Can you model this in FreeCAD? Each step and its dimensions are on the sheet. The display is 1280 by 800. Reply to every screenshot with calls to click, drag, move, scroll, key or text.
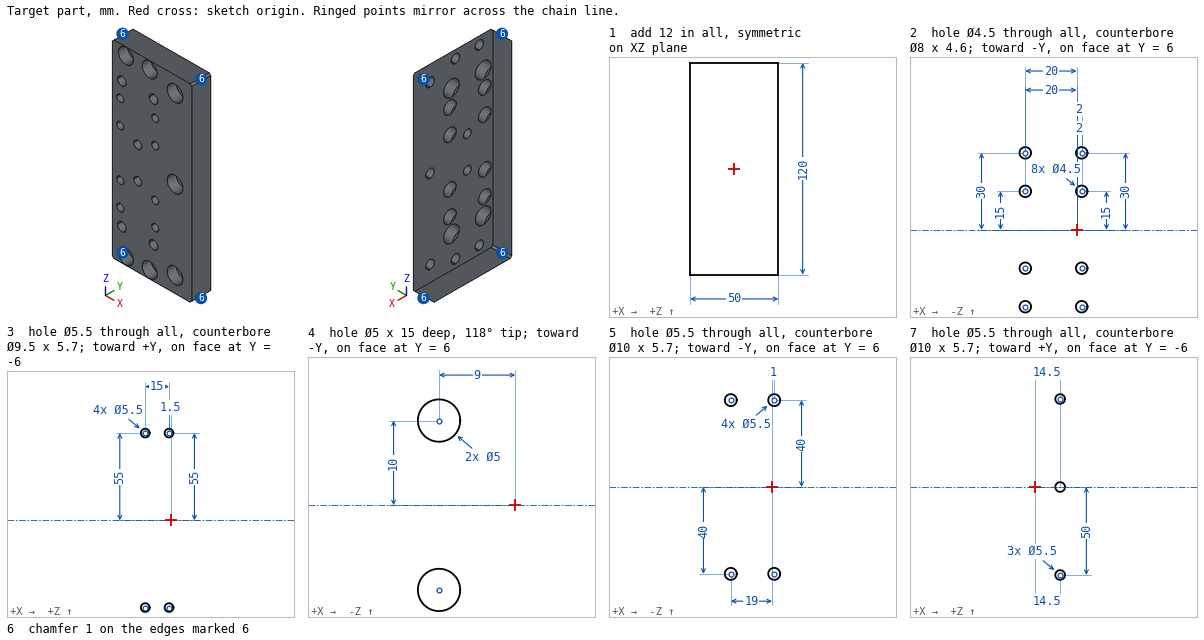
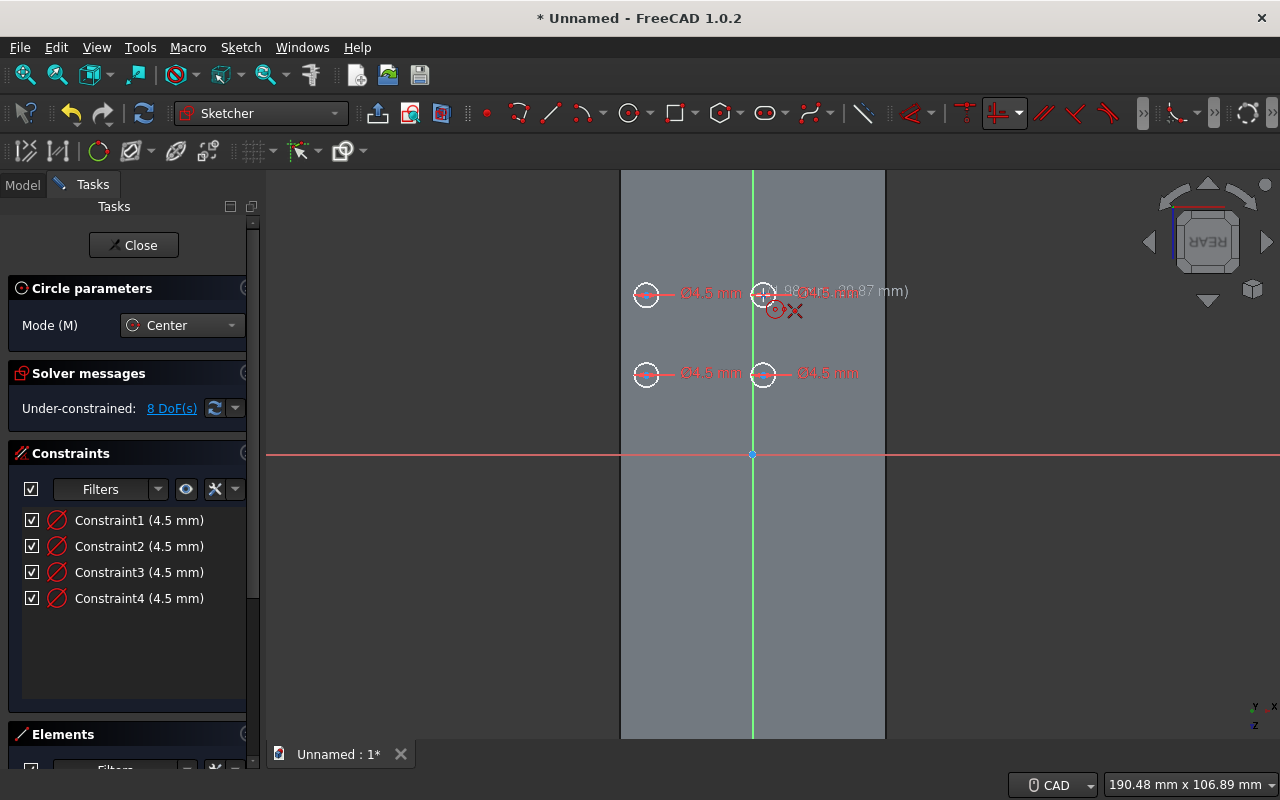
scroll(646, 534, up, 4)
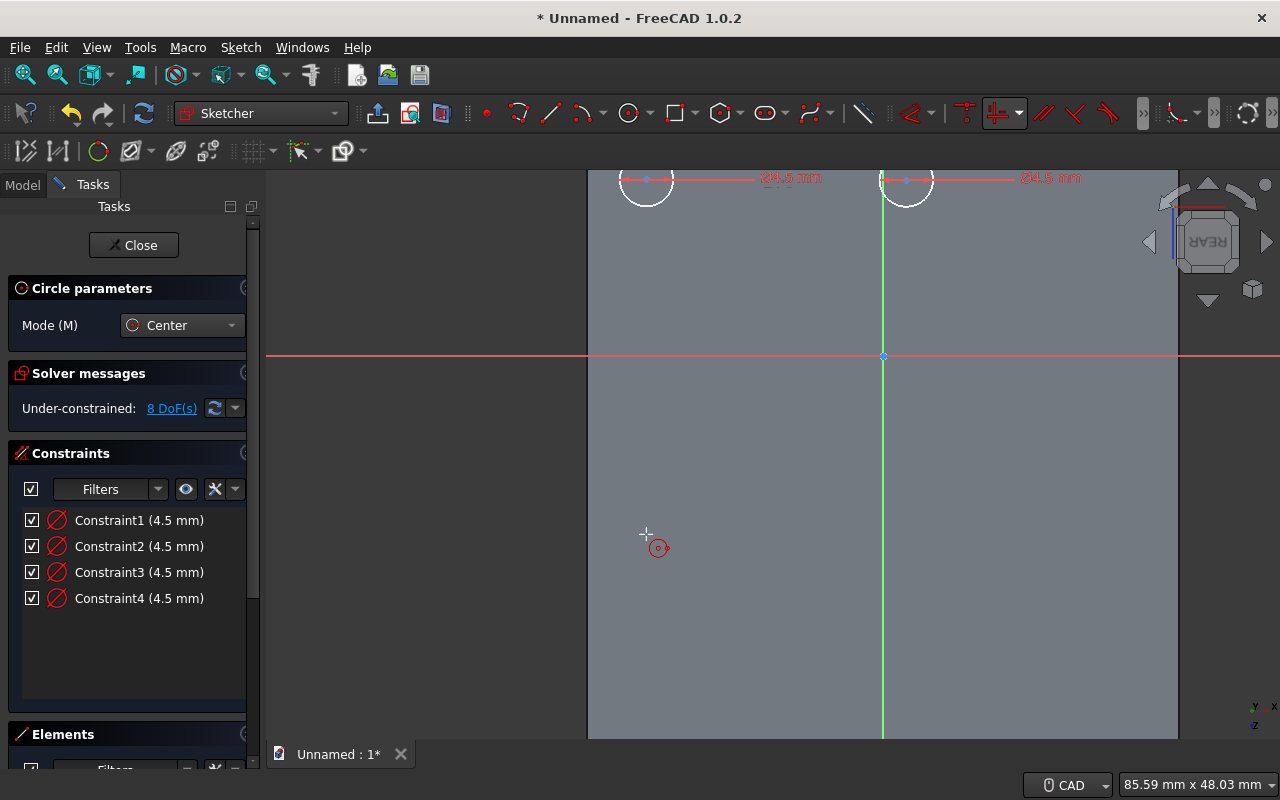
click(646, 534)
move(665, 515)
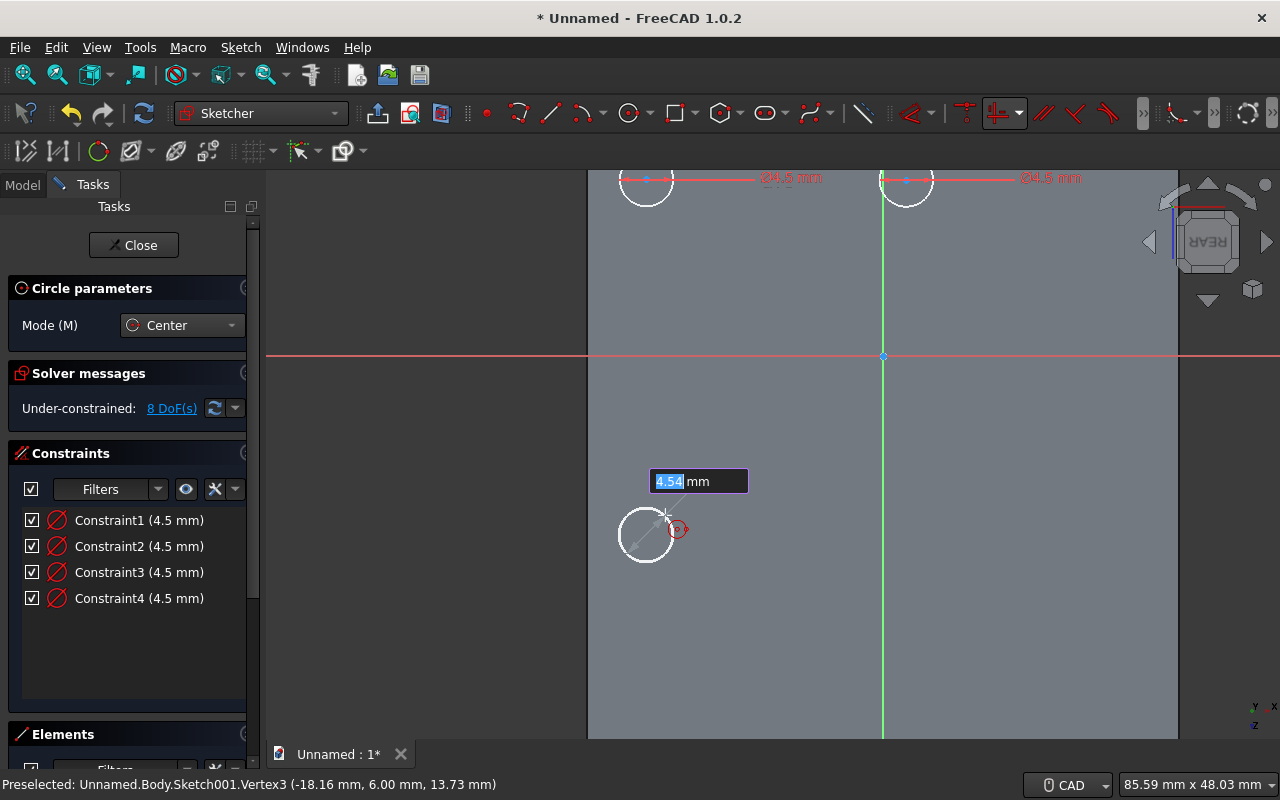
text(4.5)
key(Return)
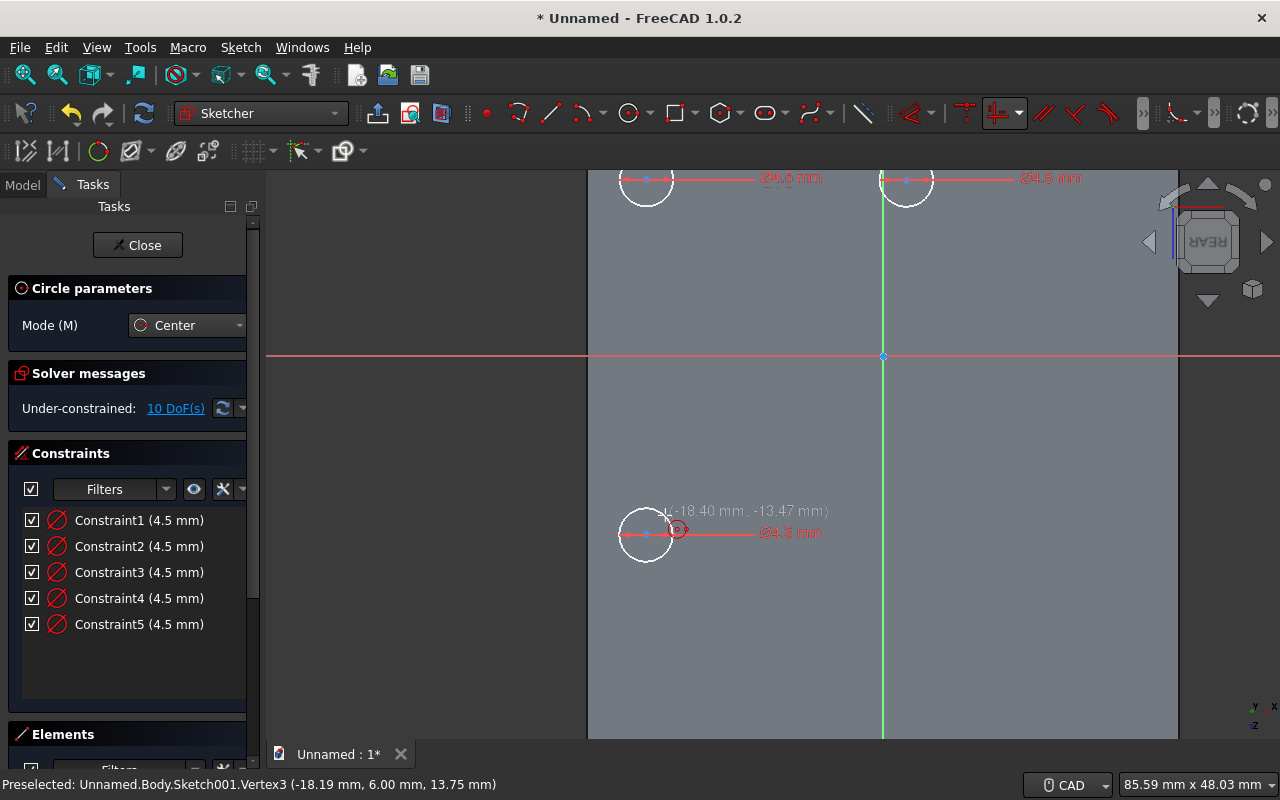
scroll(646, 535, down, 4)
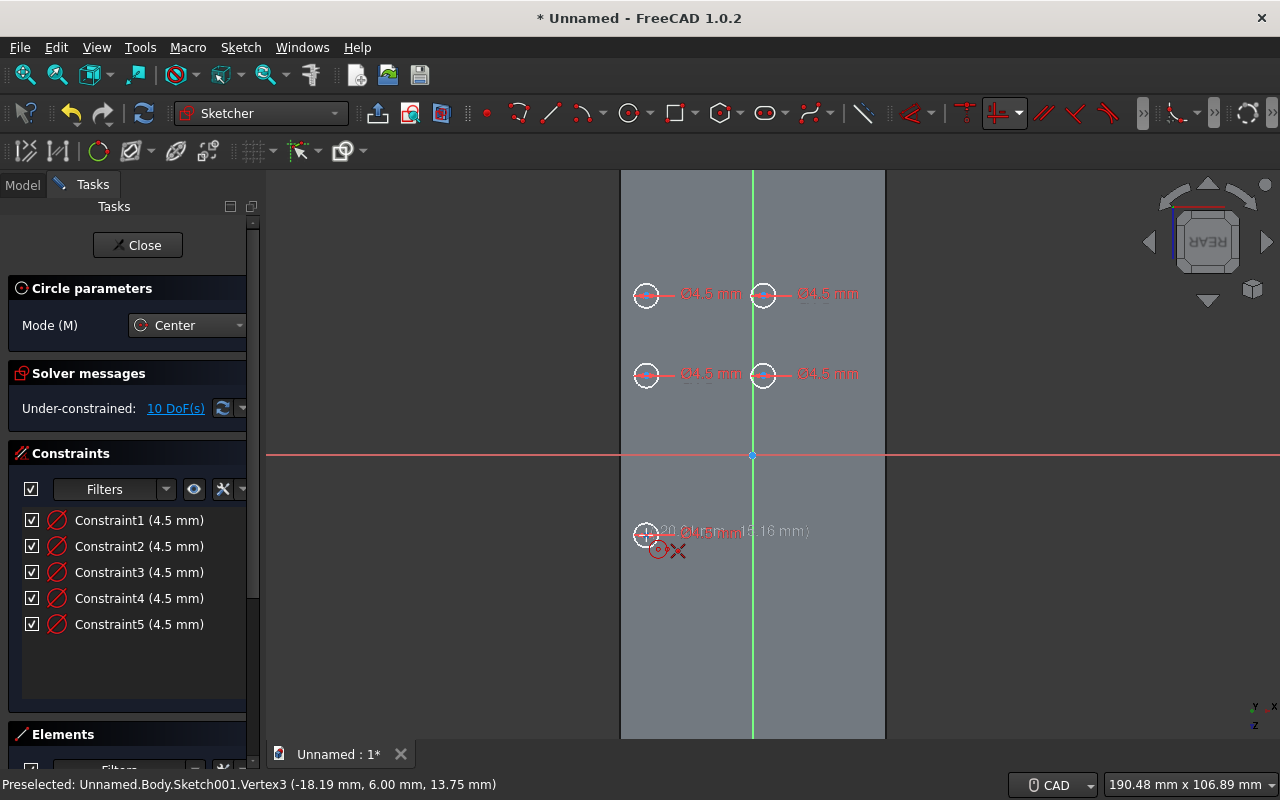
scroll(763, 615, up, 4)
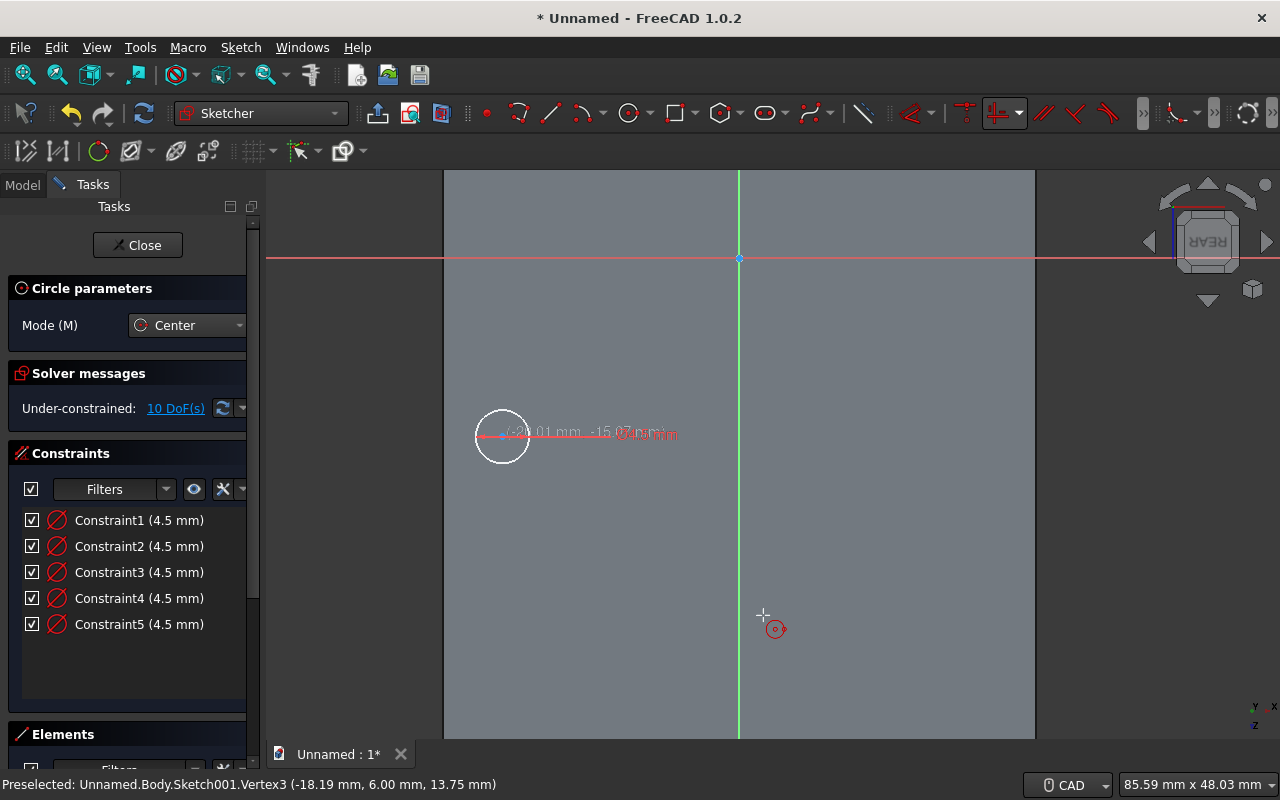
click(763, 614)
move(782, 595)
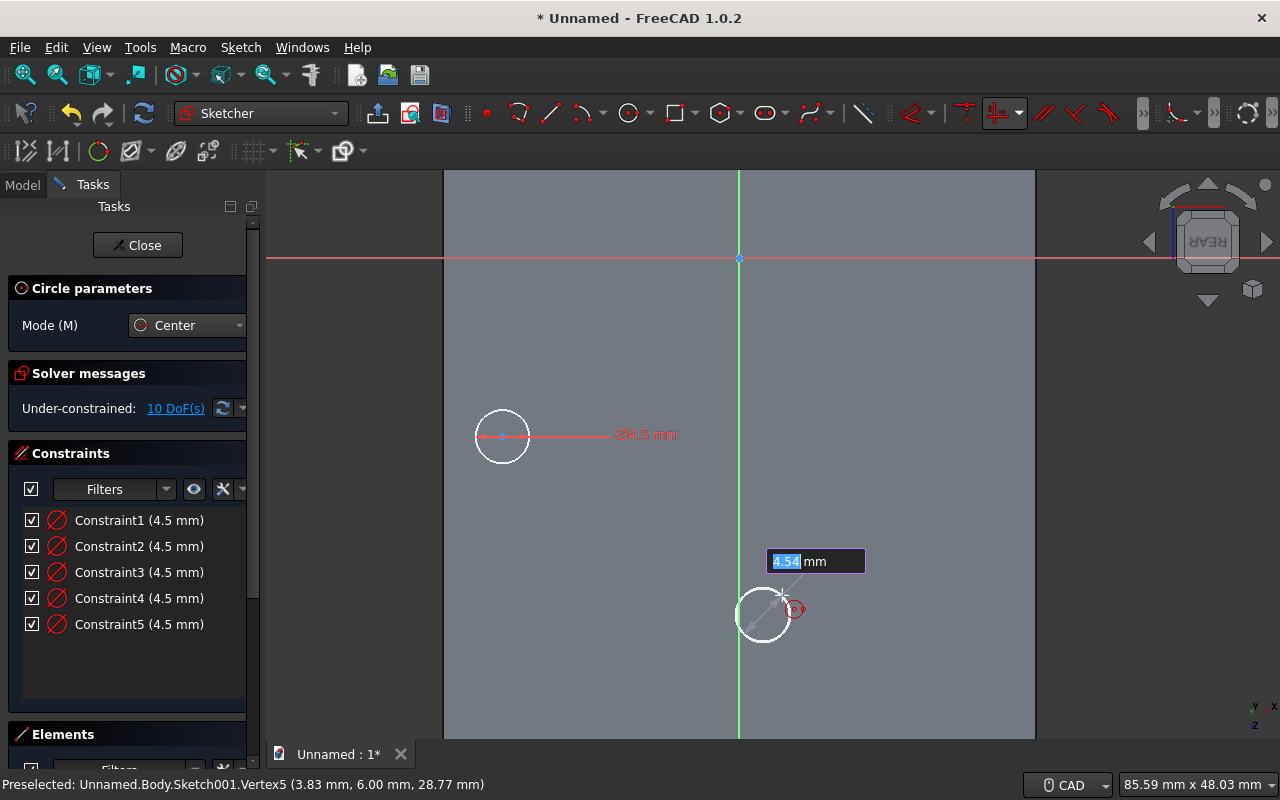
text(4.5)
key(Return)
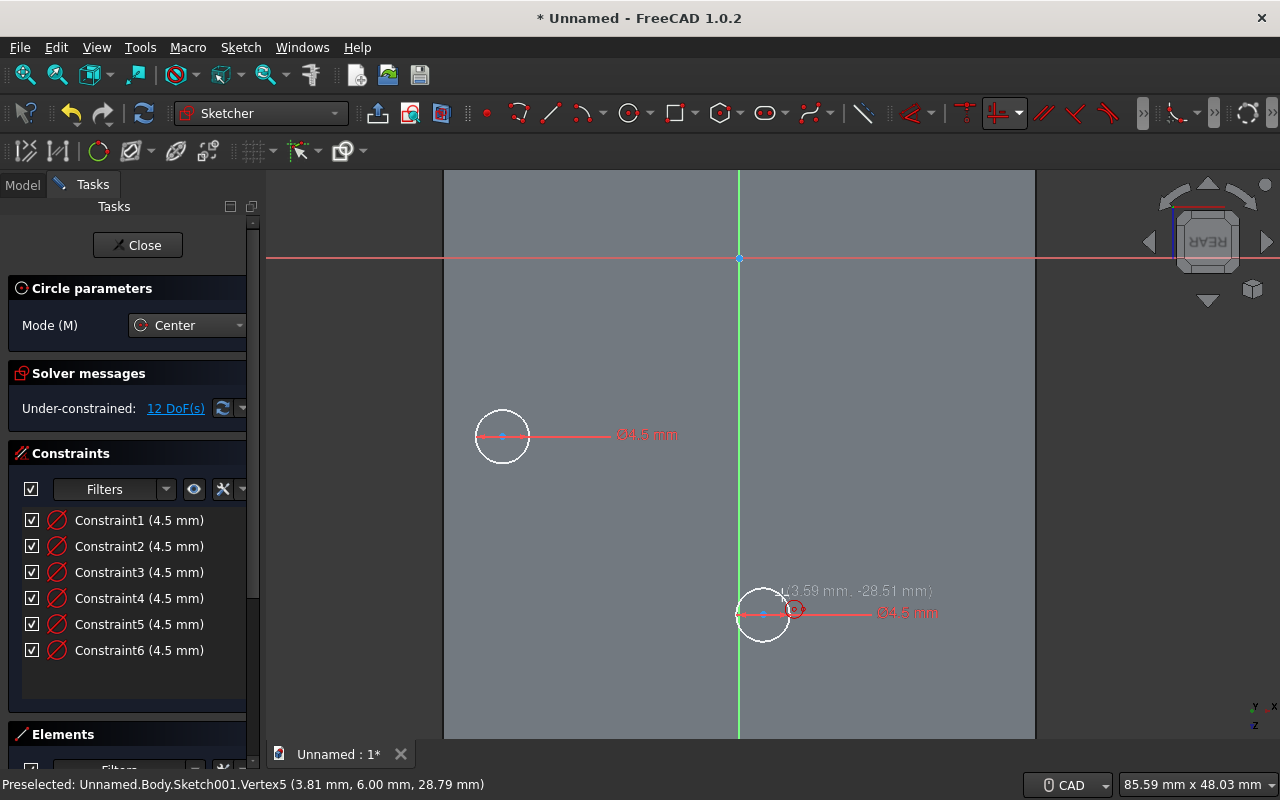
click(503, 614)
move(521, 595)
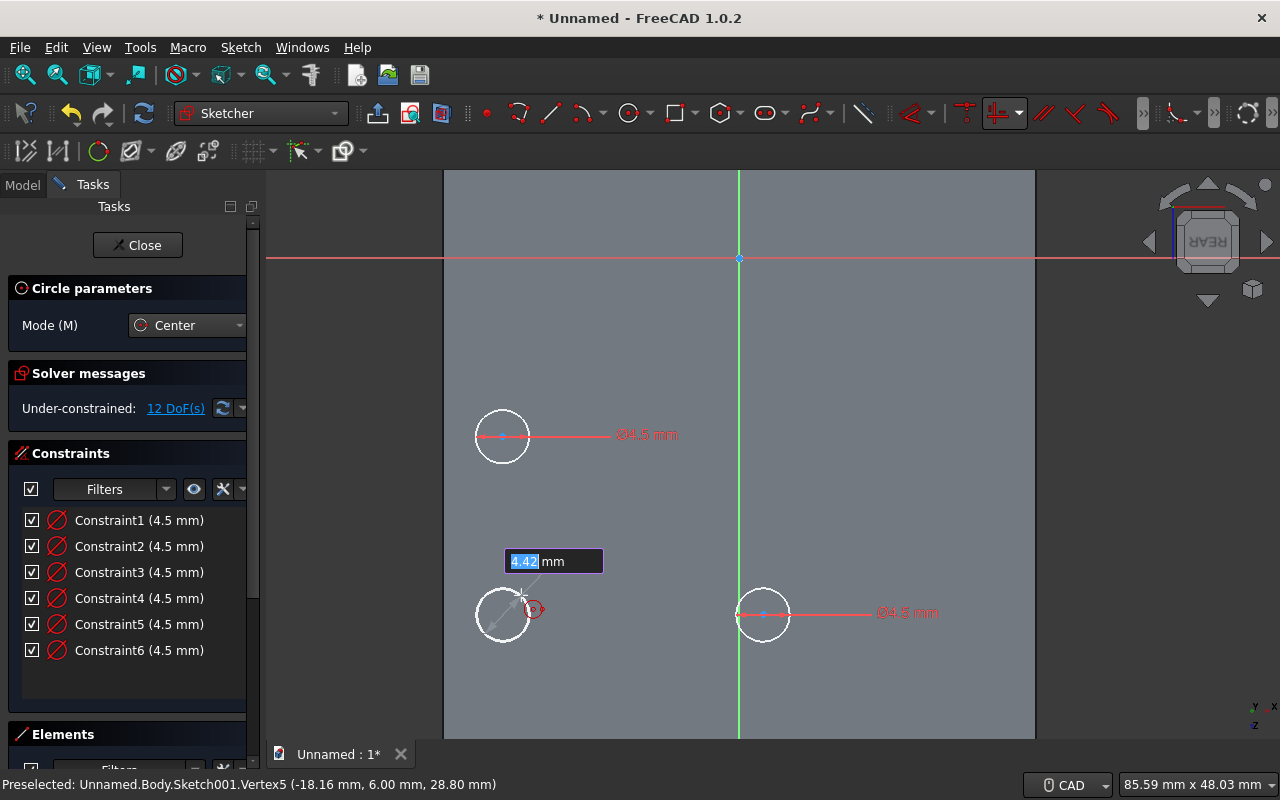
text(4.5)
key(Return)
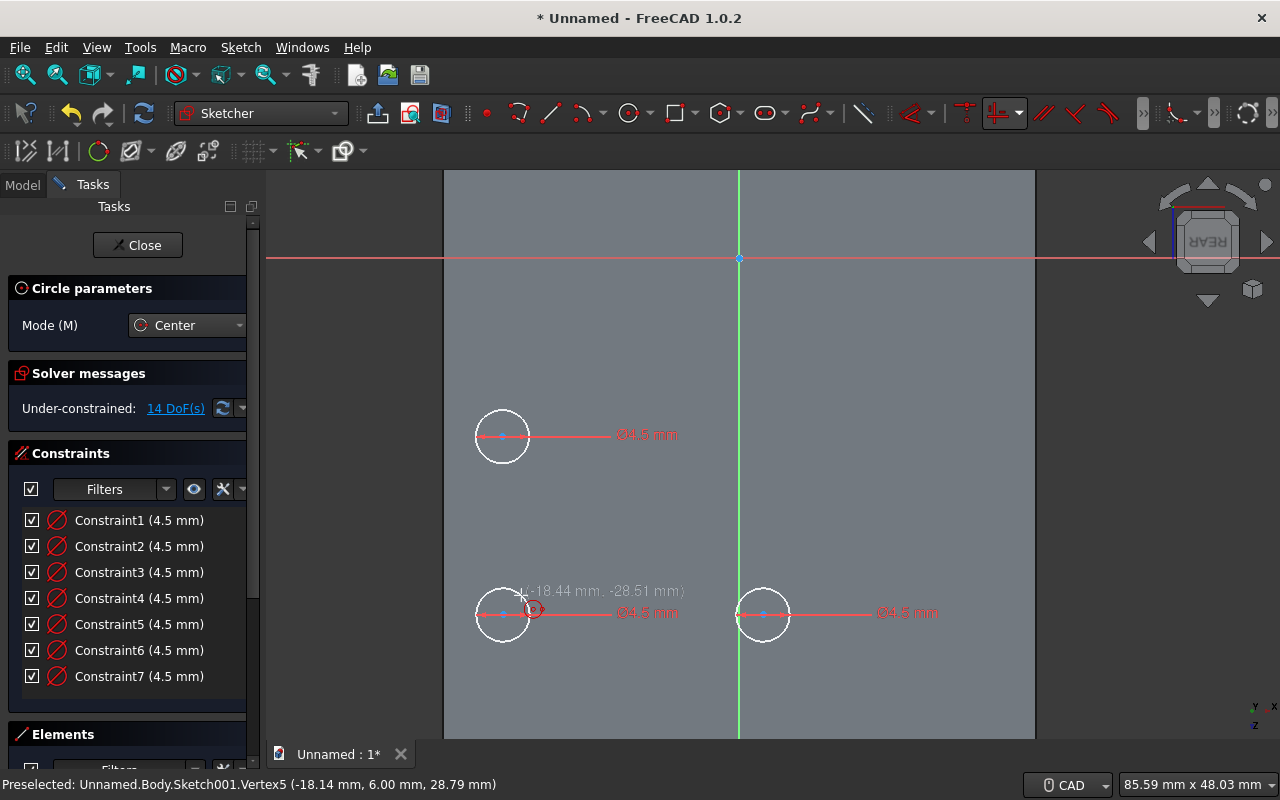
click(763, 436)
move(782, 417)